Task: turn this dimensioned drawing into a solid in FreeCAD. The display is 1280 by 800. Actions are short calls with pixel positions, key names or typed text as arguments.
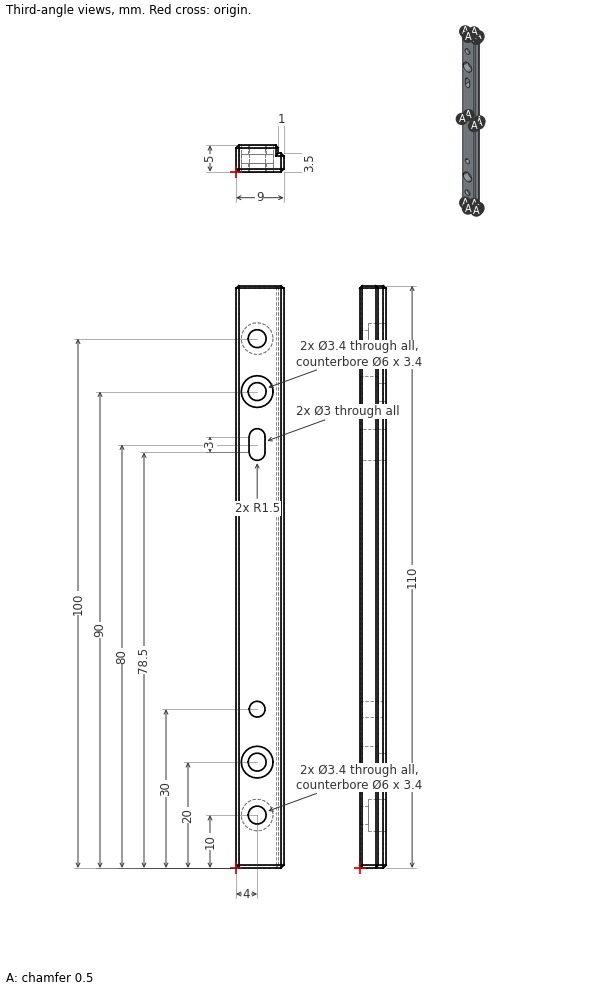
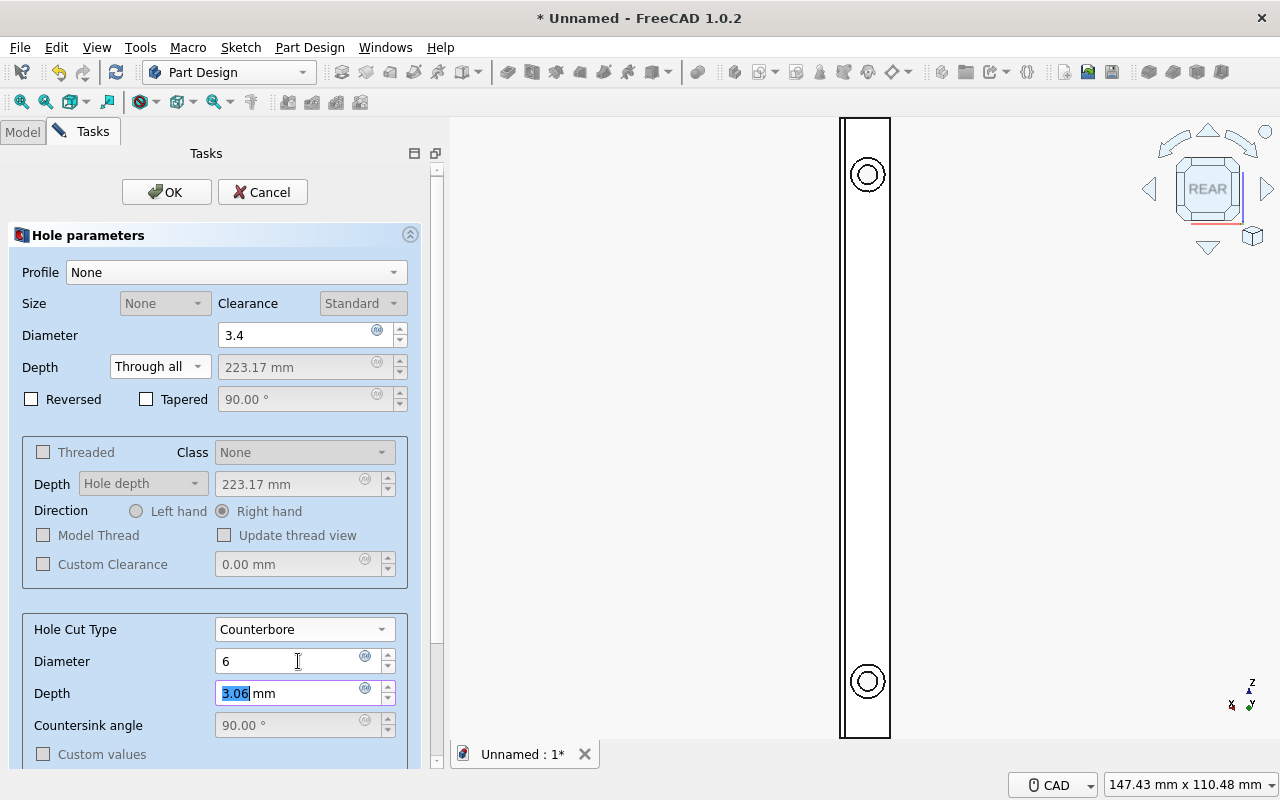
text(3.4)
key(Tab)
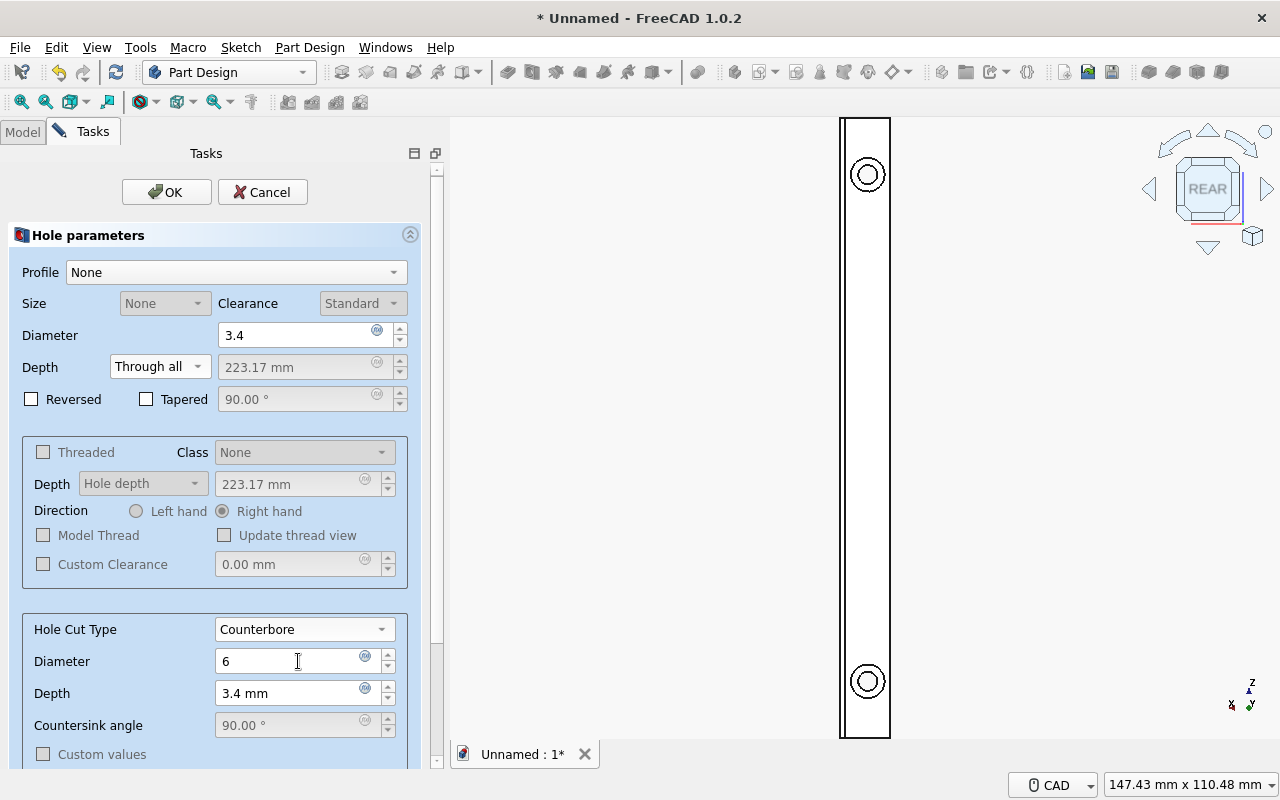
click(167, 192)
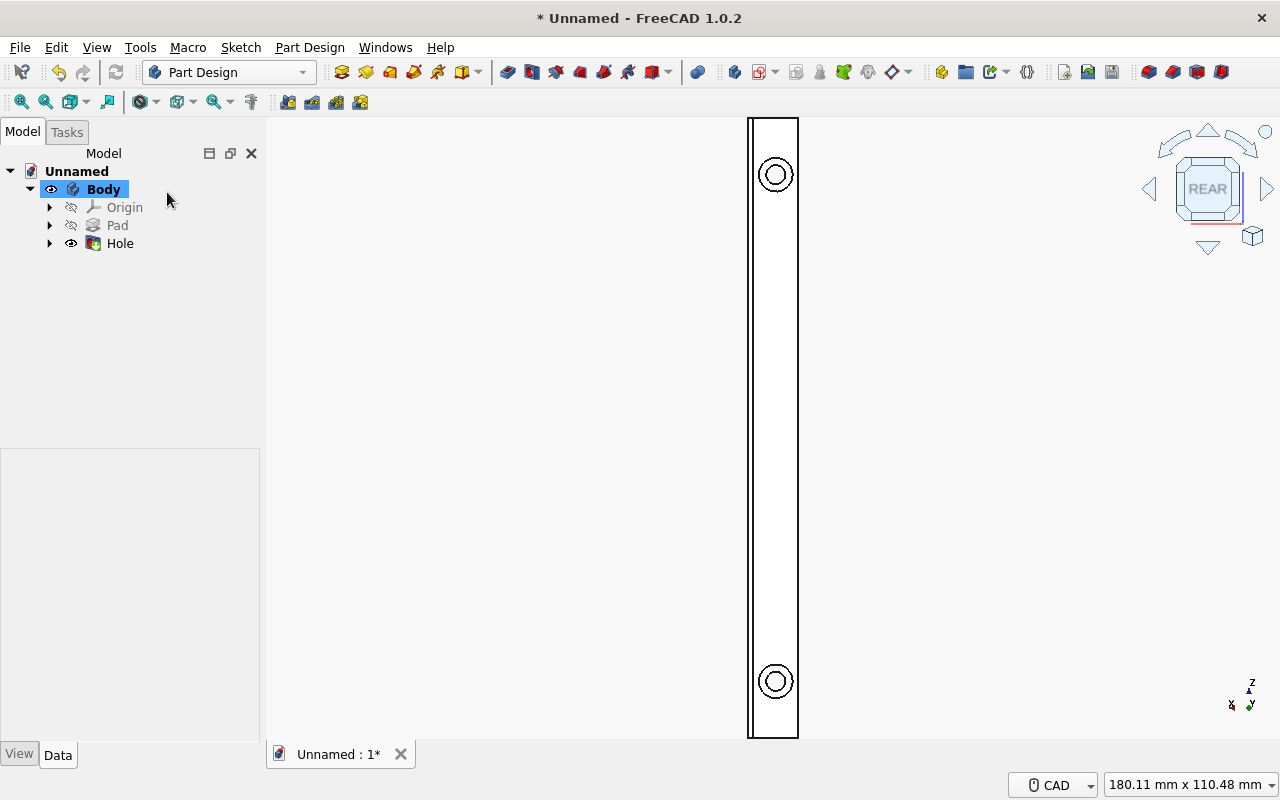
key(0)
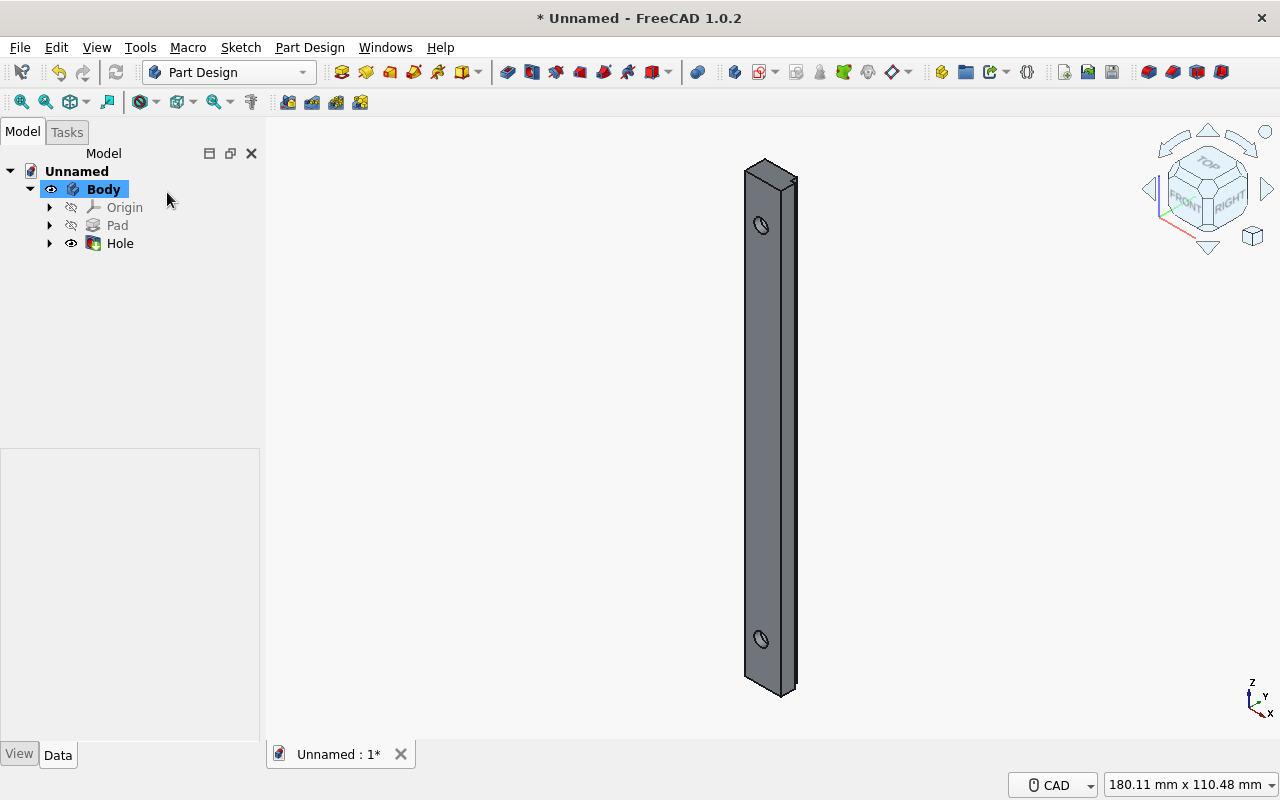
click(763, 288)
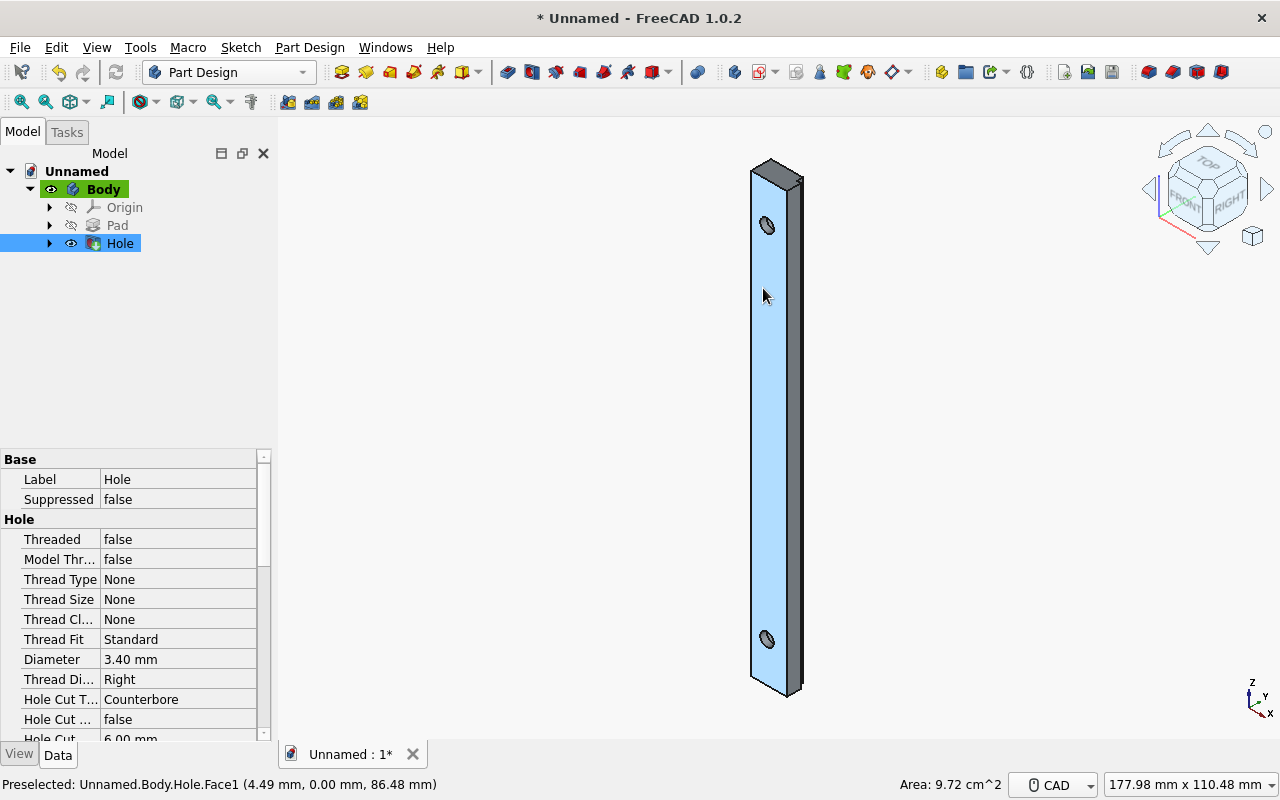
click(760, 72)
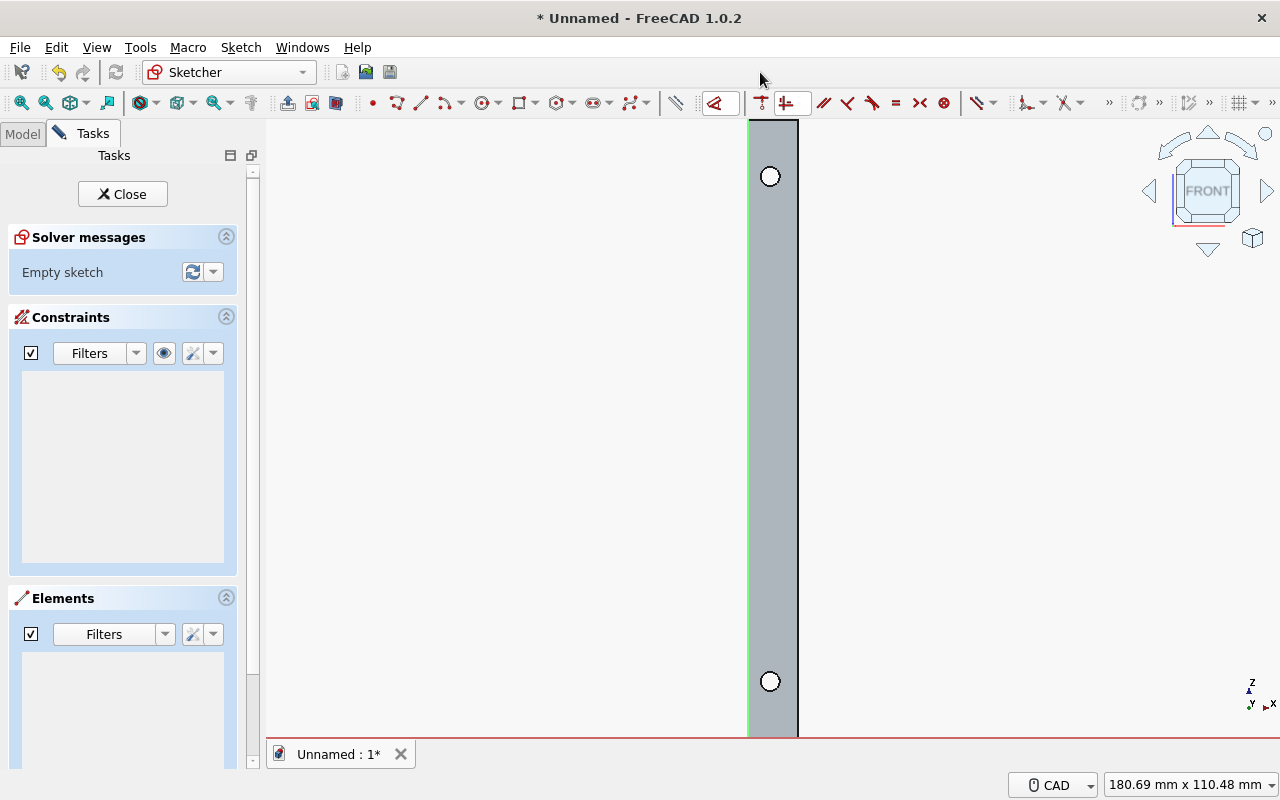
scroll(437, 197, down, 1)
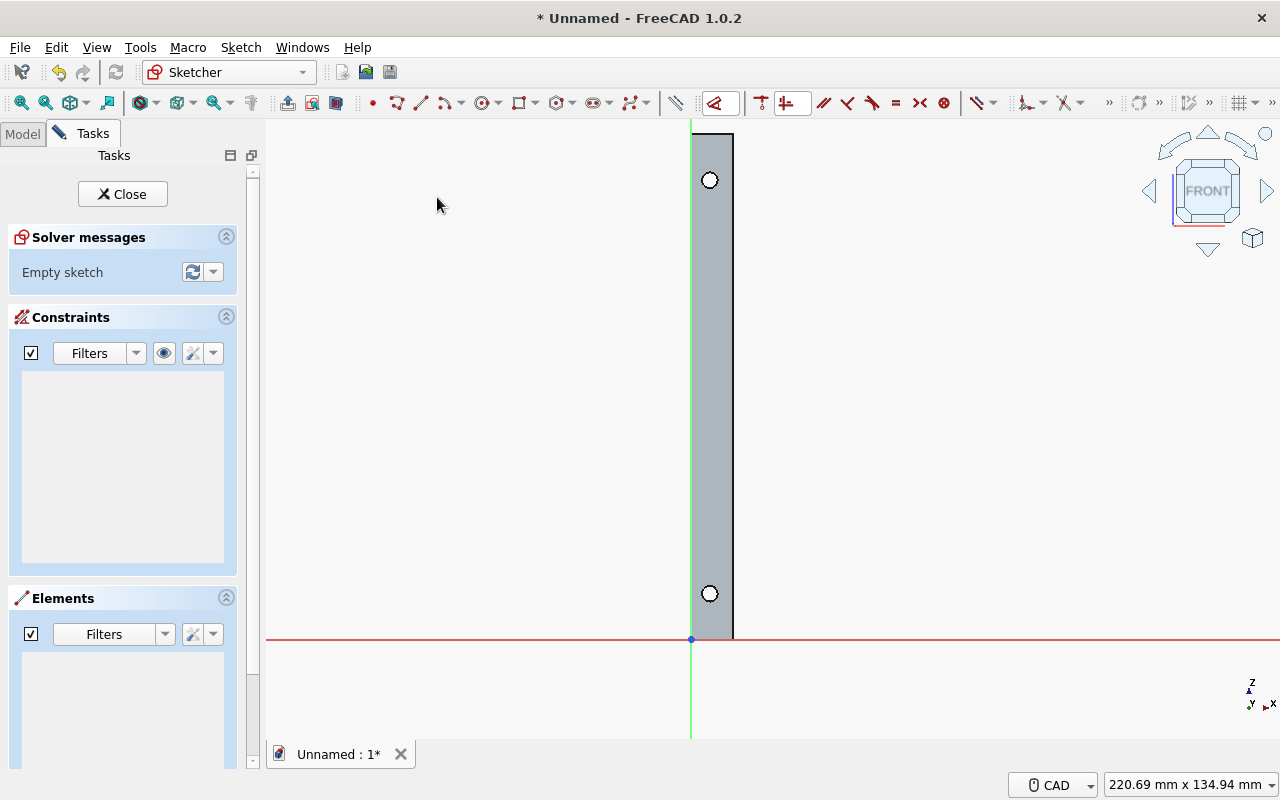
key(g)
key(c)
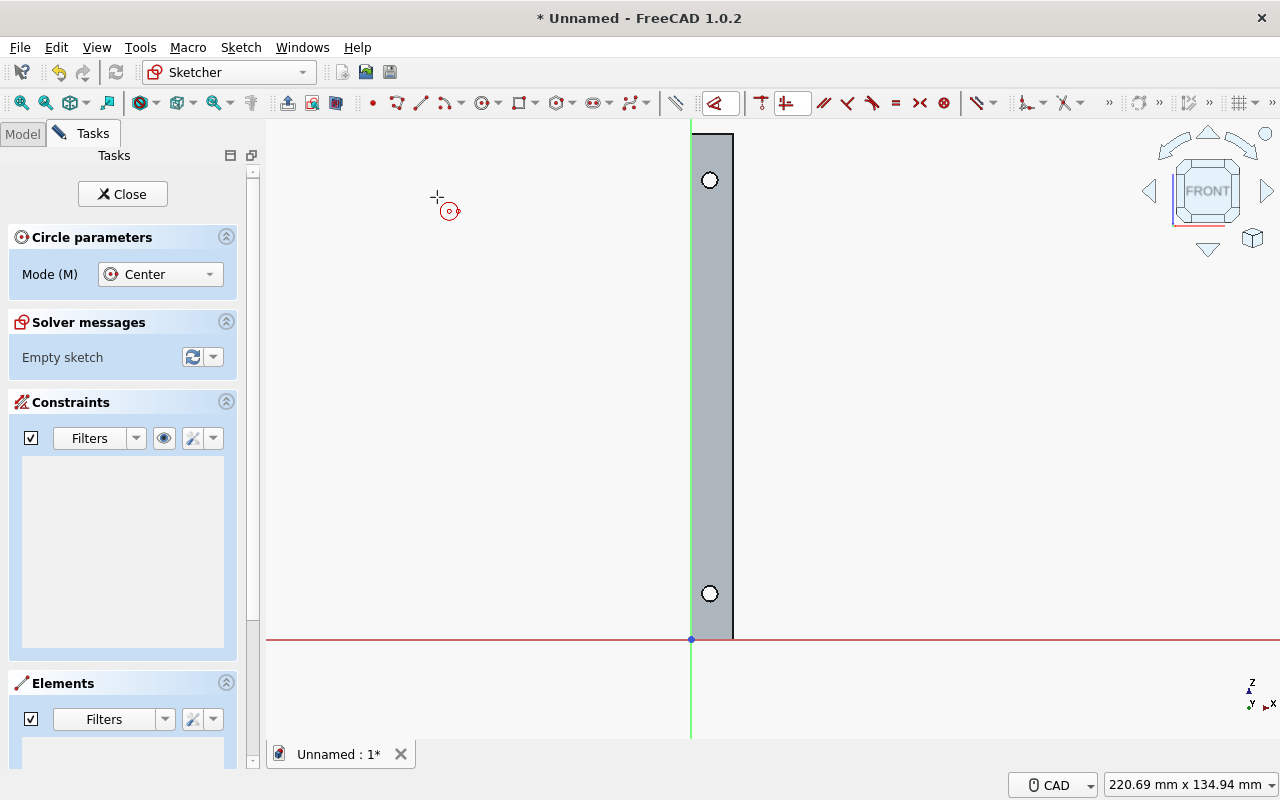
scroll(710, 226, up, 6)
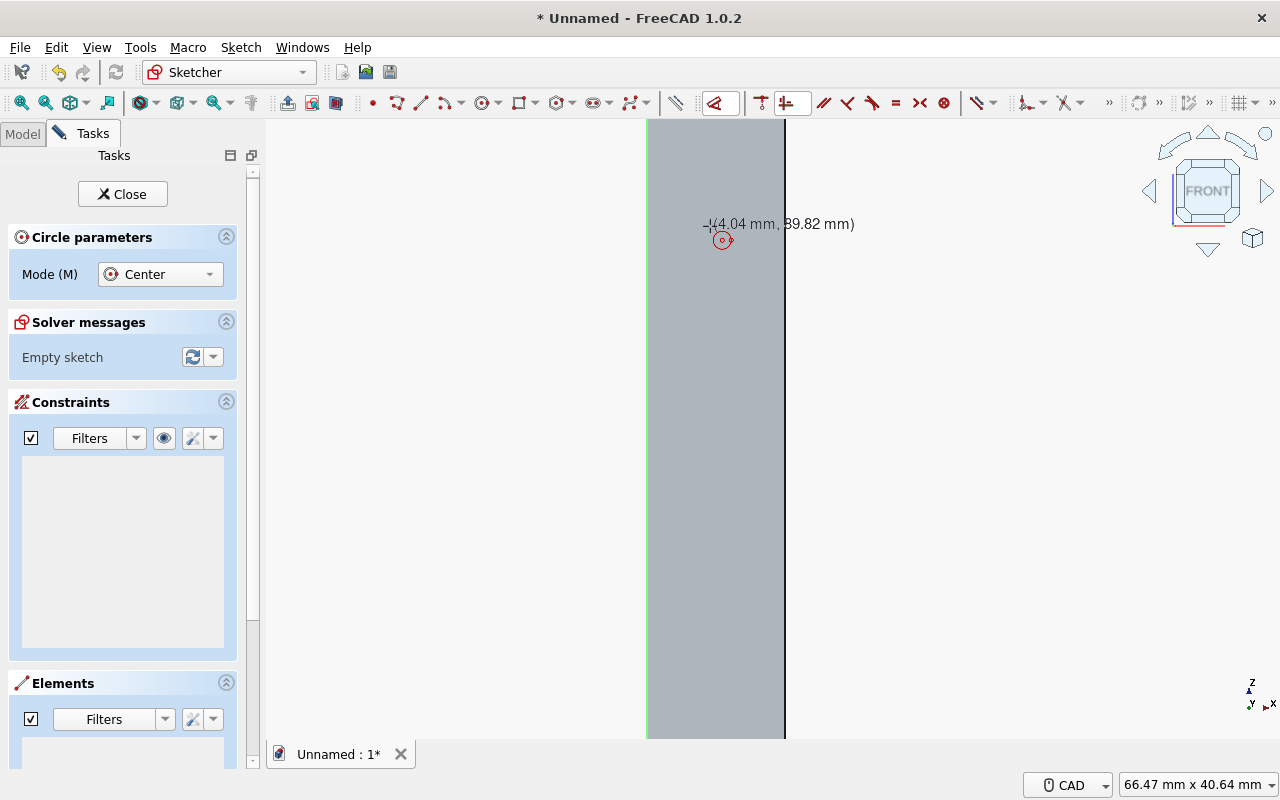
click(708, 226)
click(727, 208)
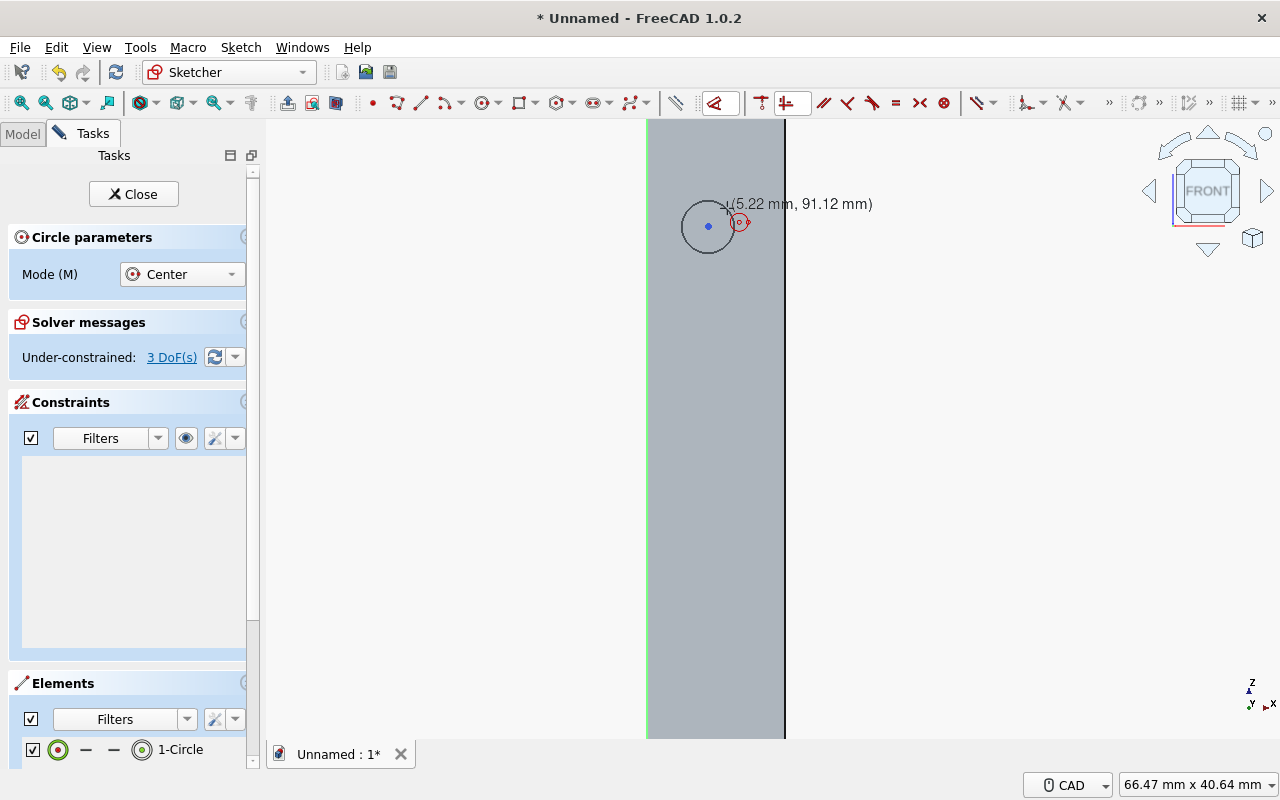
scroll(710, 226, down, 6)